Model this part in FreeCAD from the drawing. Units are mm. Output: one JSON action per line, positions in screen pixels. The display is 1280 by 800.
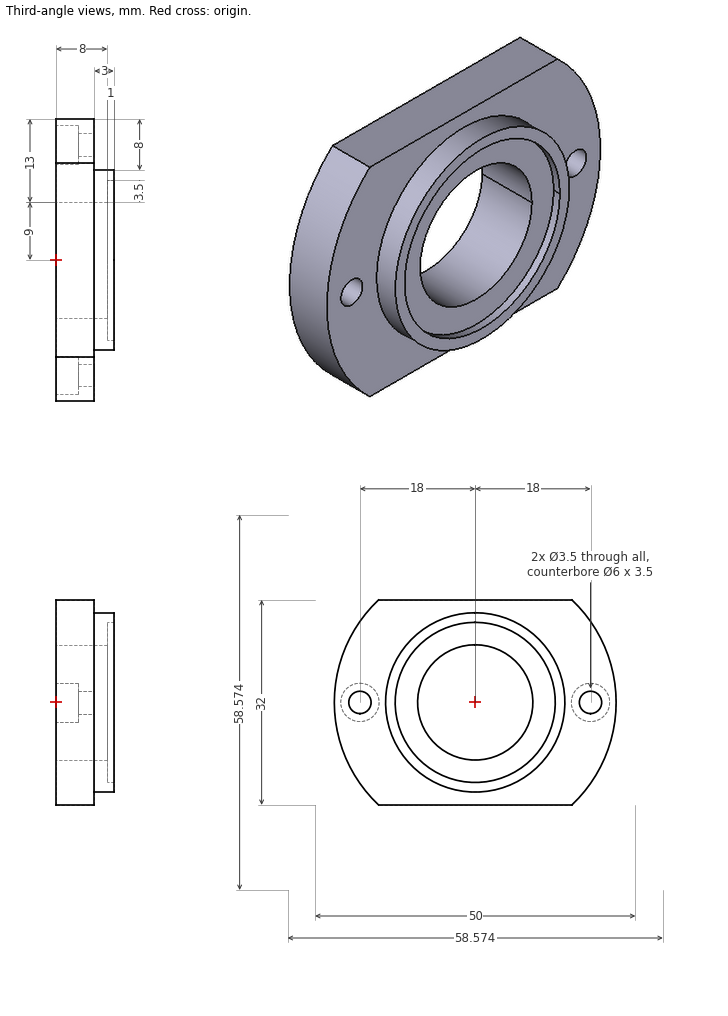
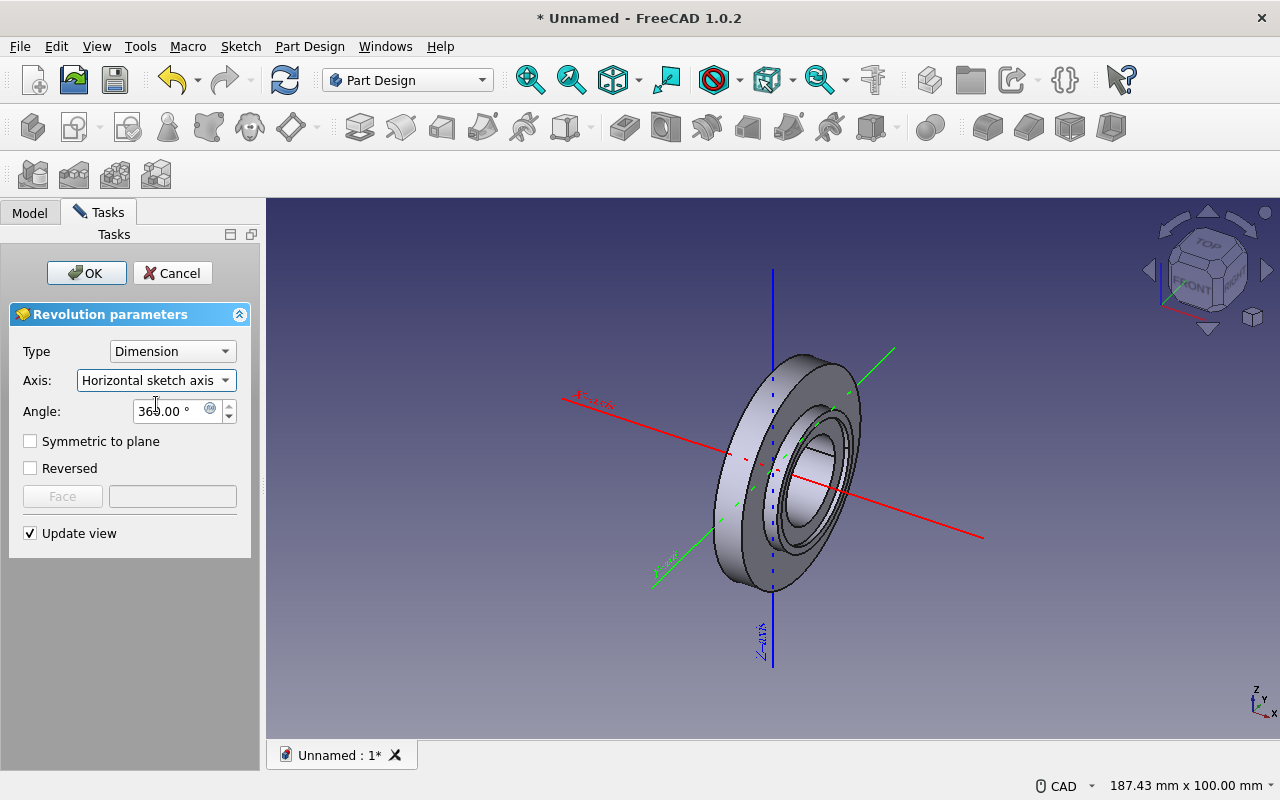
{"action": "left_click", "coordinate": [87, 273]}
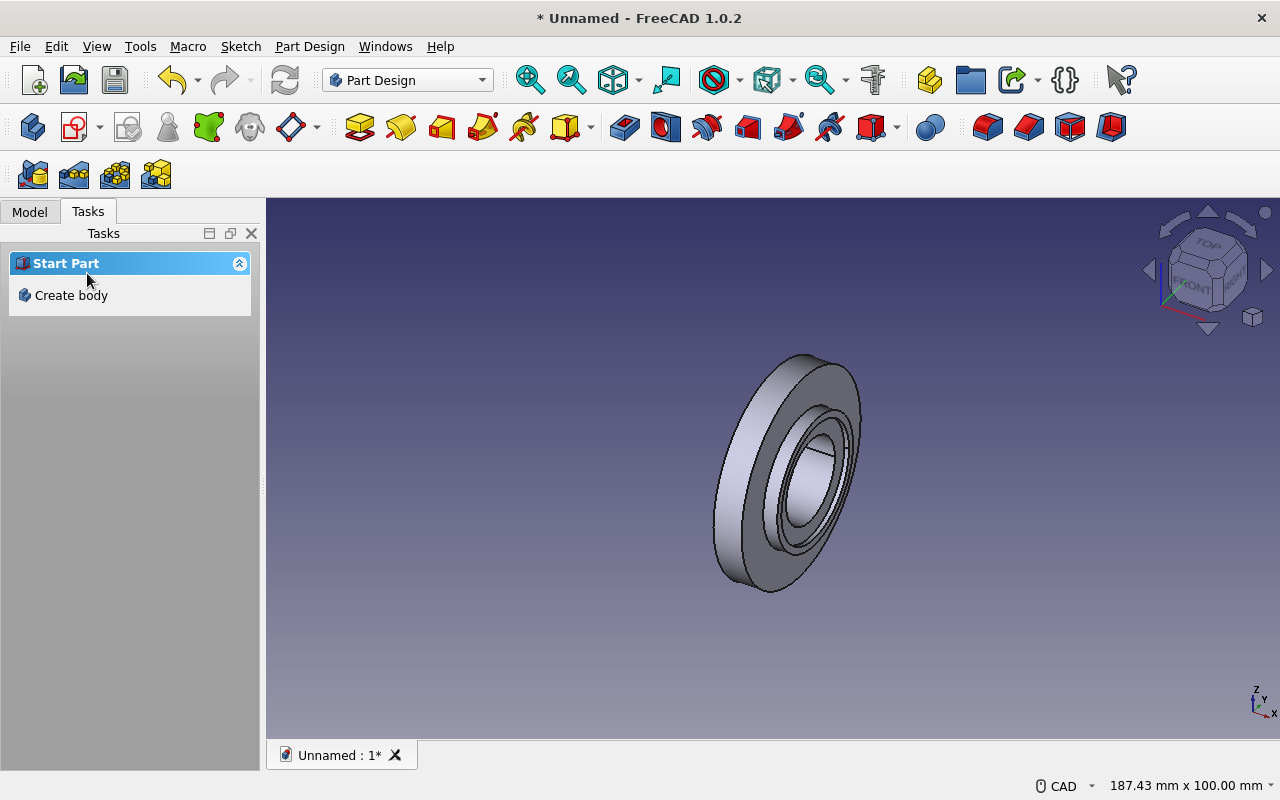
{"action": "key", "text": "6"}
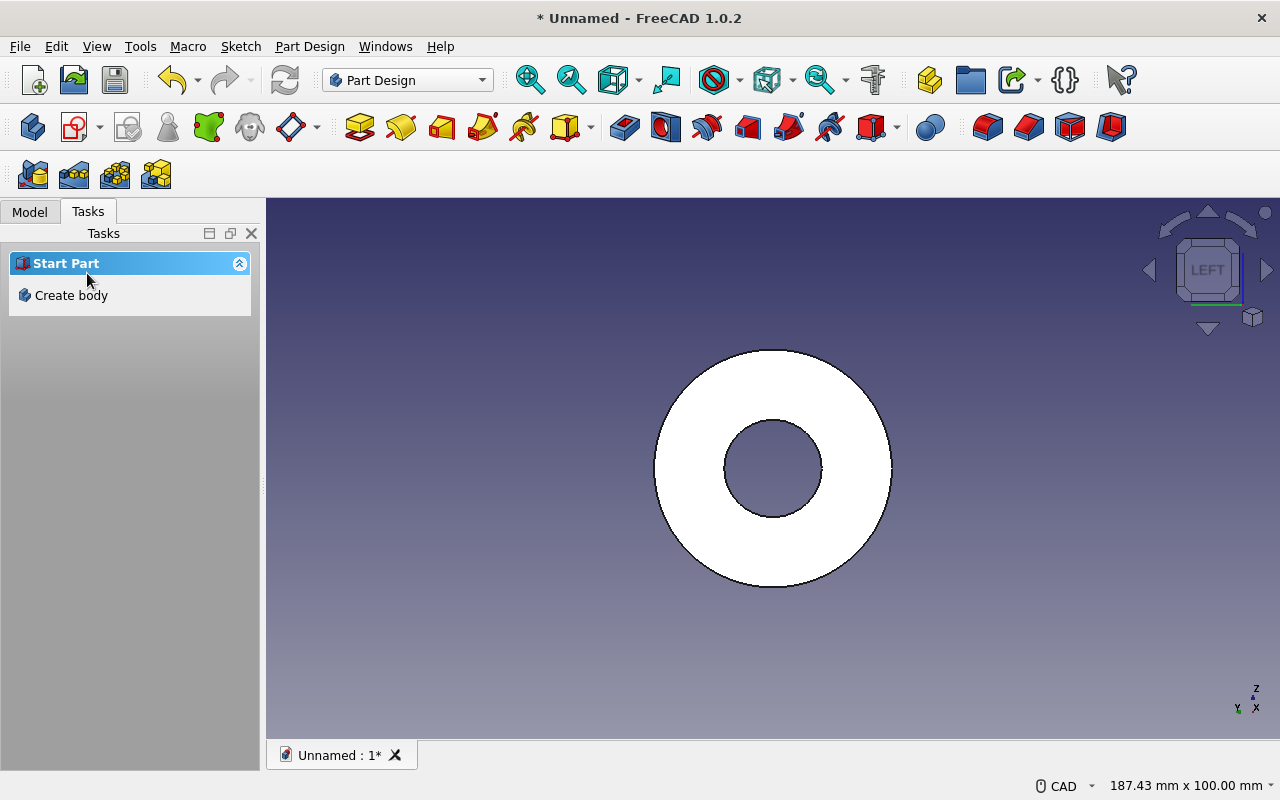
{"action": "left_click", "coordinate": [531, 80]}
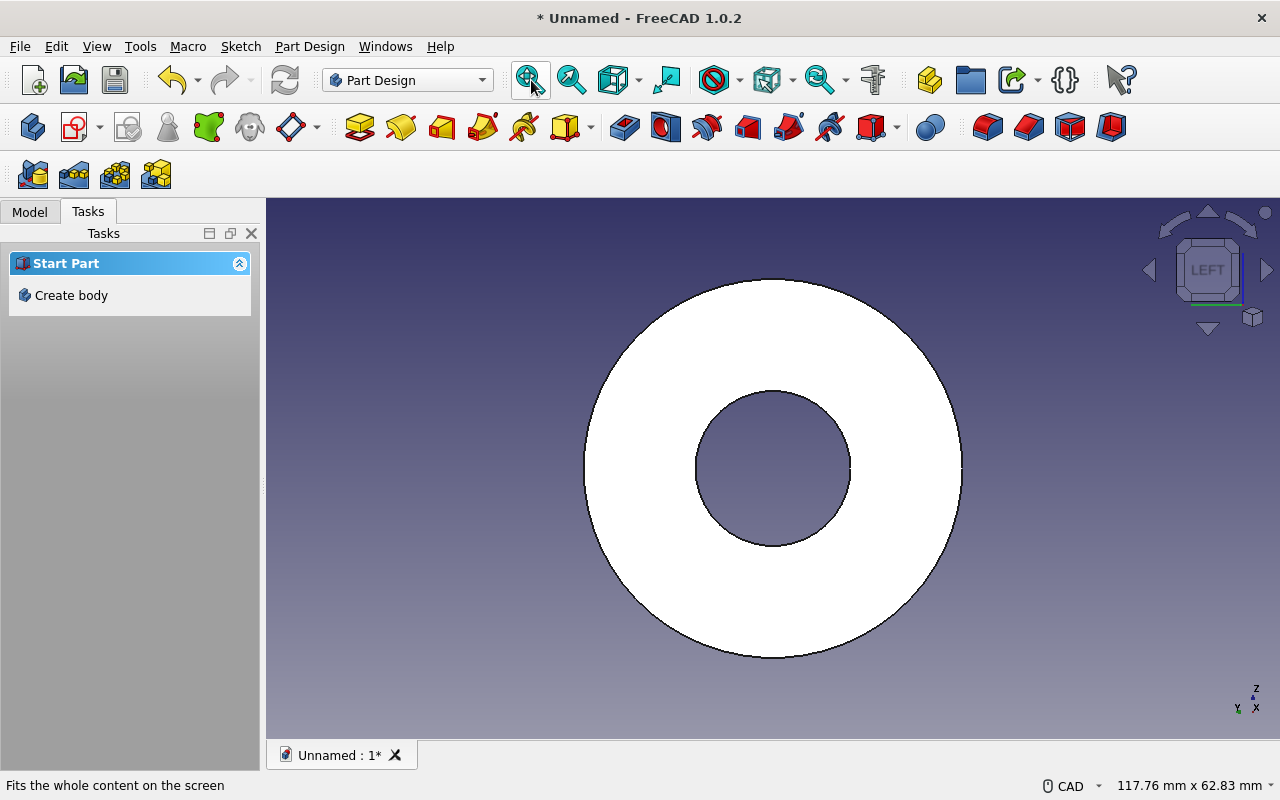
{"action": "left_click", "coordinate": [827, 576]}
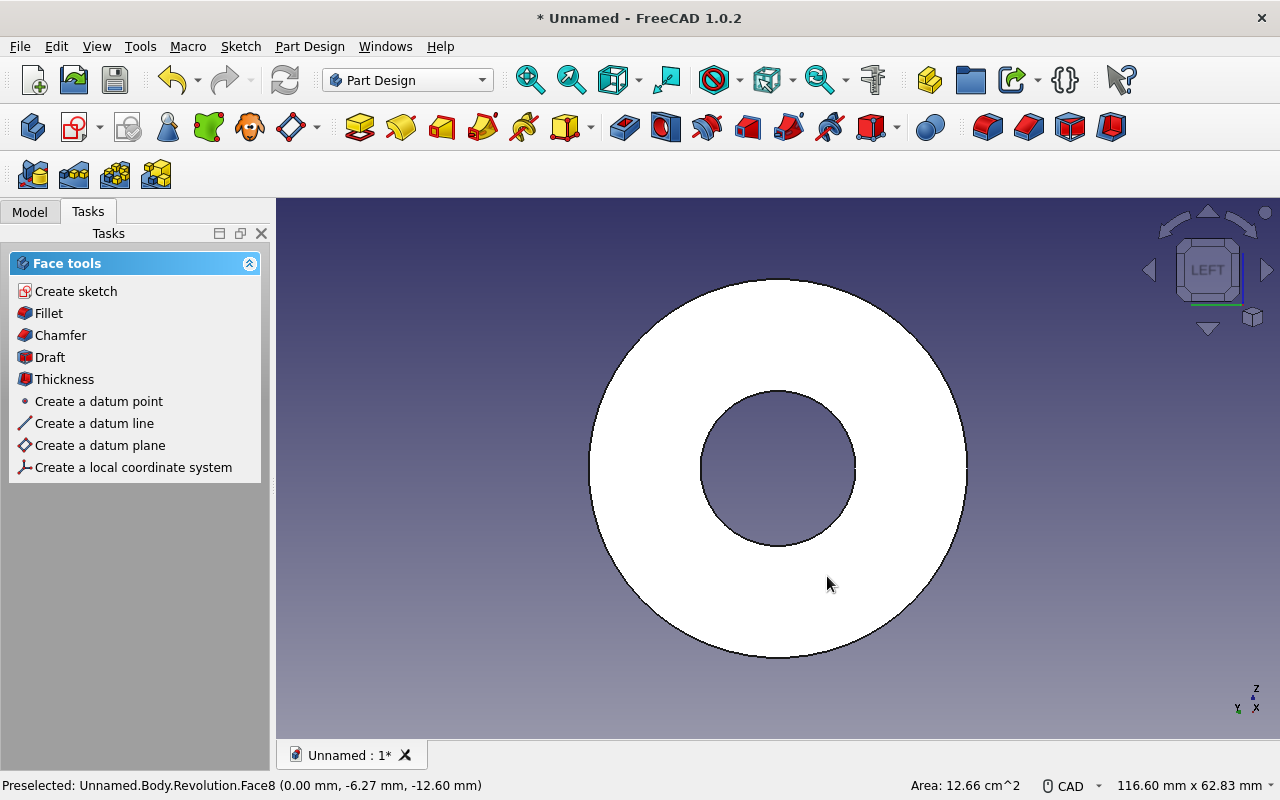
{"action": "left_click", "coordinate": [74, 128]}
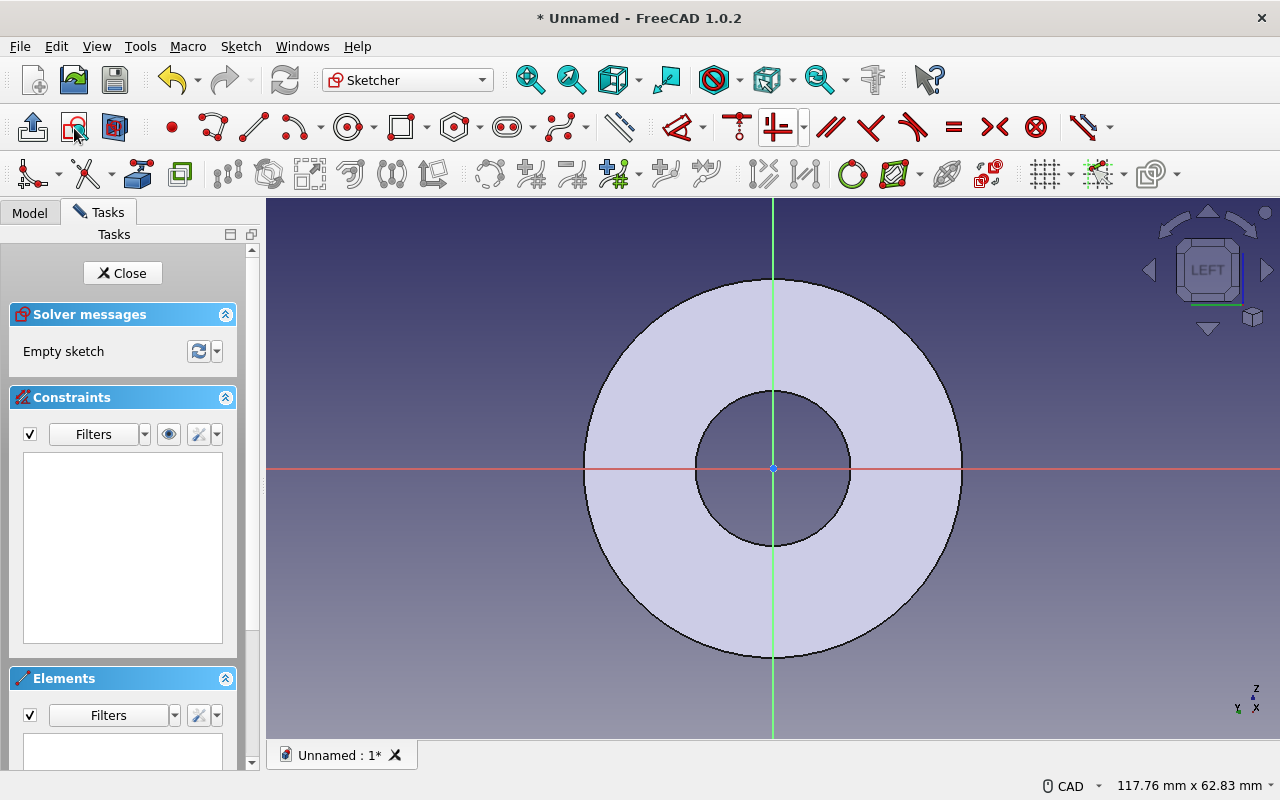
{"action": "scroll", "coordinate": [565, 468], "scroll_direction": "down", "scroll_amount": 2}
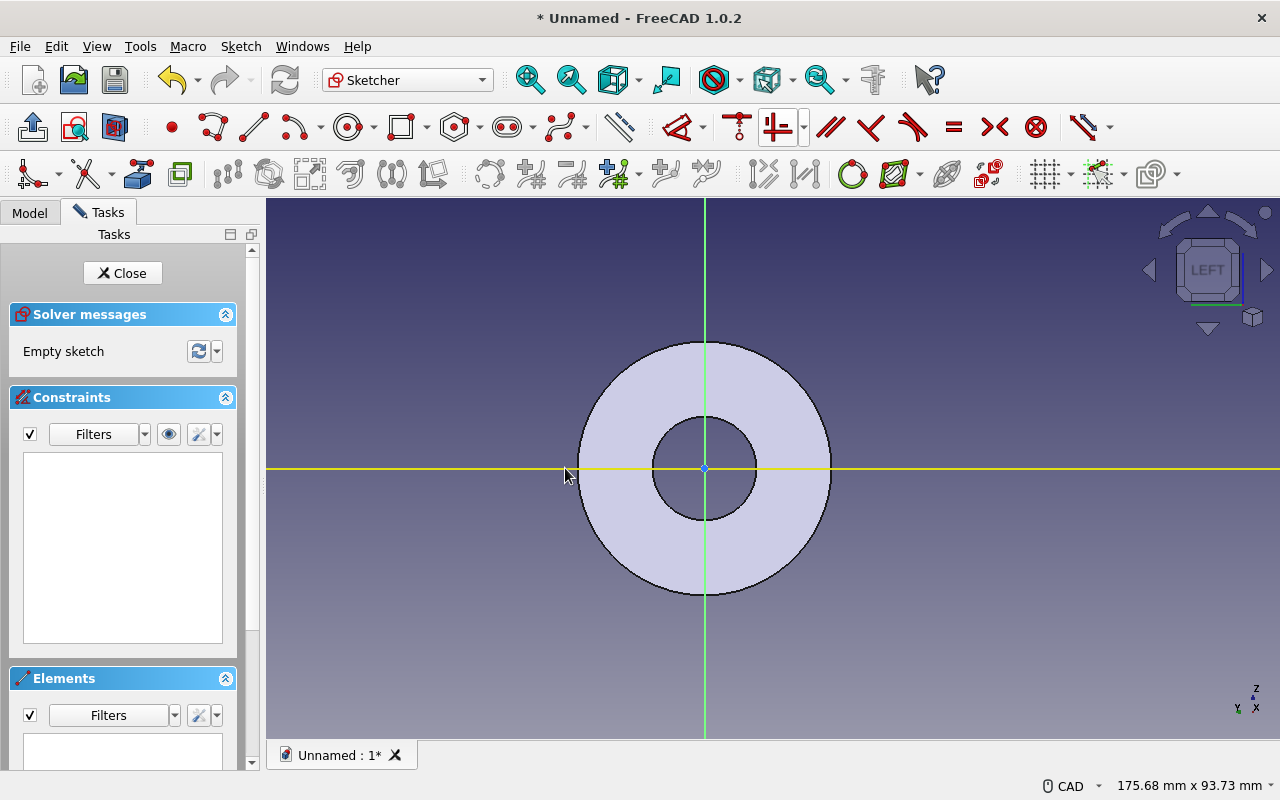
{"action": "key", "text": "g v"}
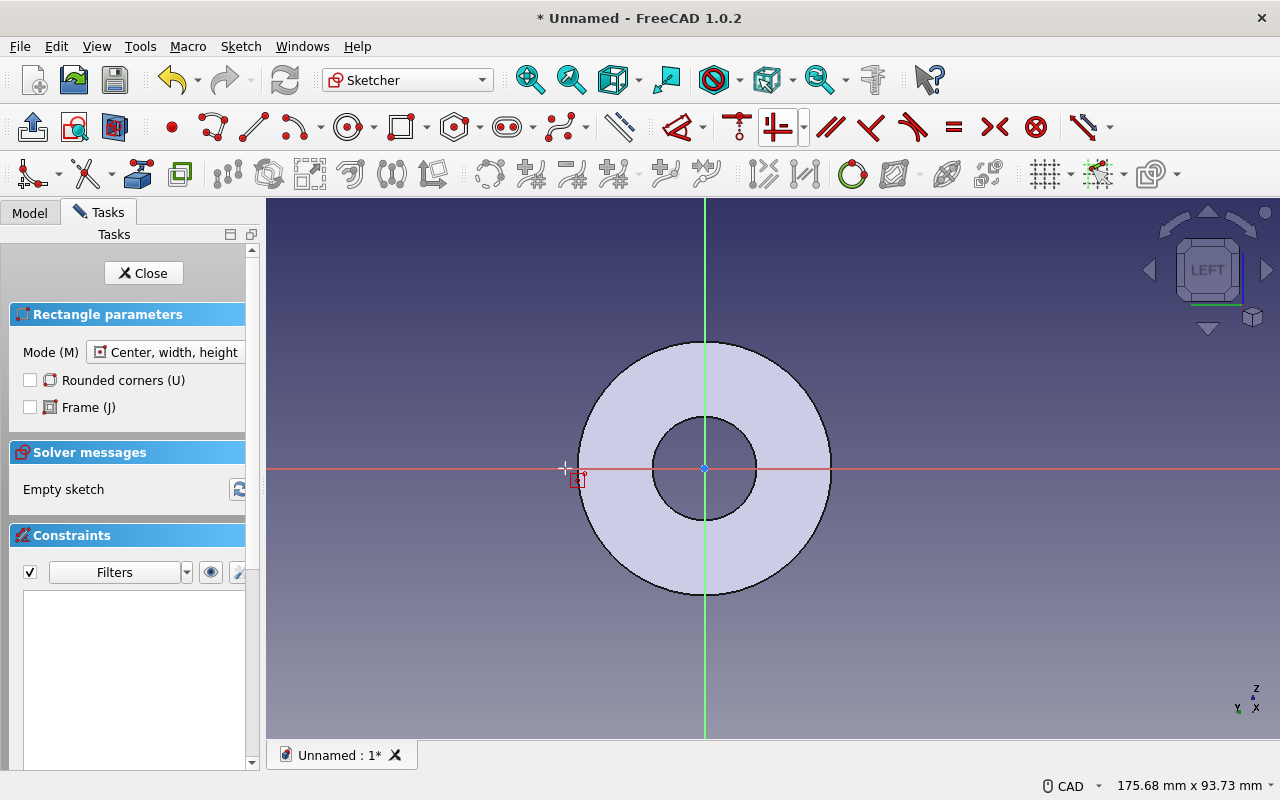
{"action": "left_click", "coordinate": [705, 468]}
{"action": "mouse_move", "coordinate": [874, 299]}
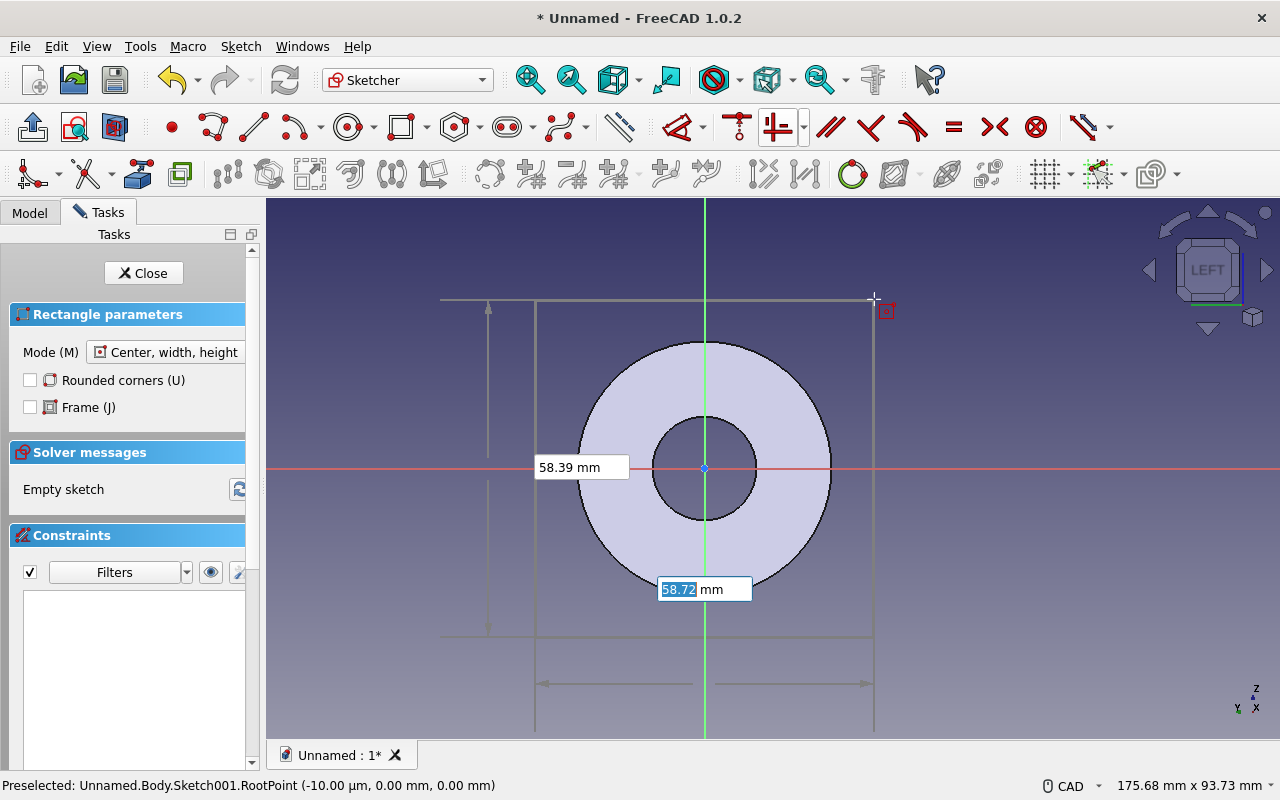
{"action": "type", "text": "58.574"}
{"action": "key", "text": "Tab"}
{"action": "type", "text": "58.574"}
{"action": "key", "text": "Return"}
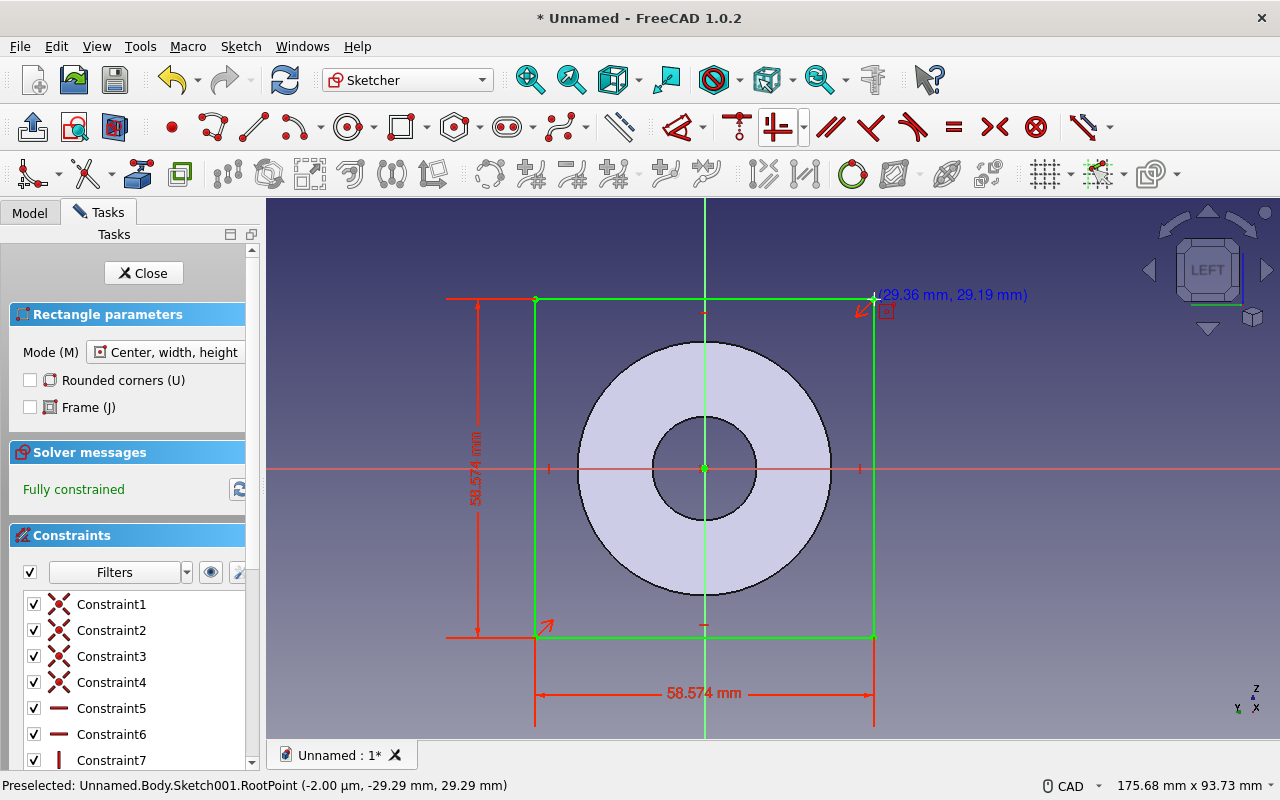
{"action": "left_click", "coordinate": [705, 468]}
{"action": "mouse_move", "coordinate": [849, 376]}